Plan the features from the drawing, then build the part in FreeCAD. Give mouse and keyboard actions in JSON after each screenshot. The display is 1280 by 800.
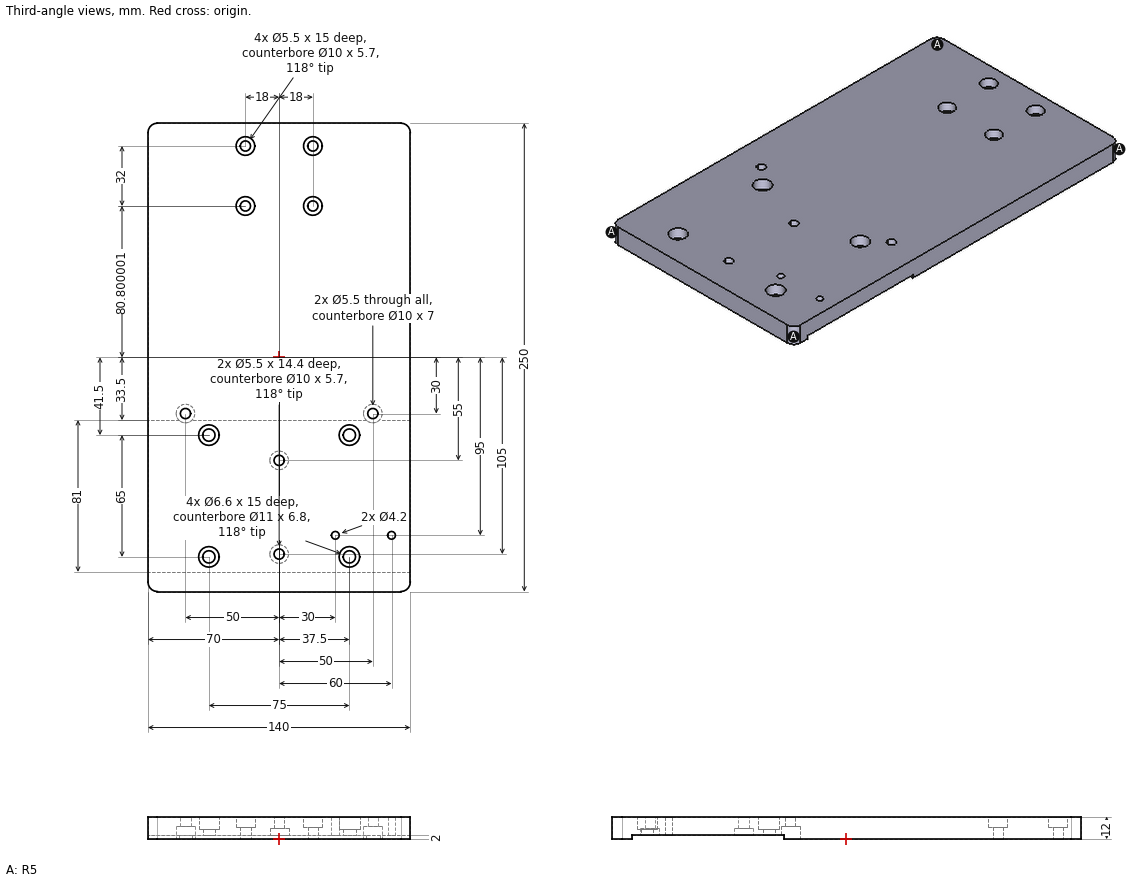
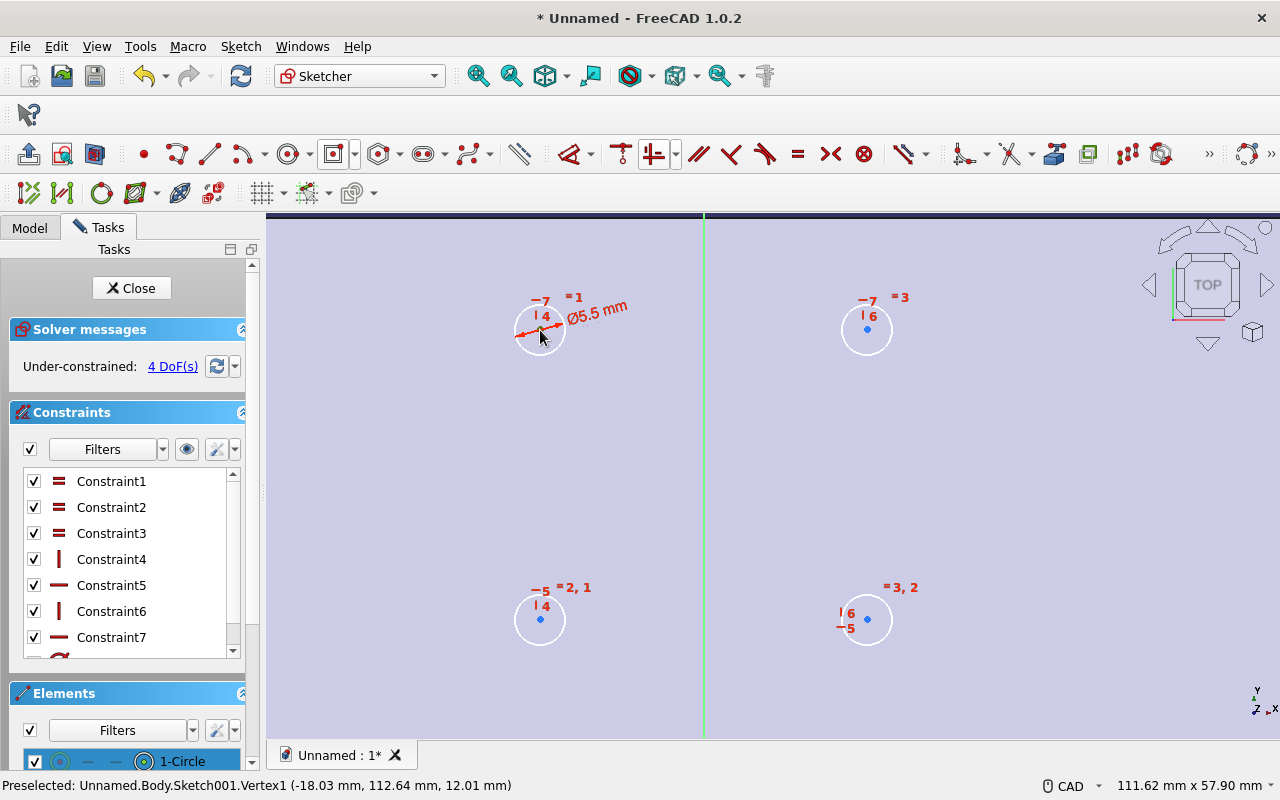
{"action": "key", "text": "l"}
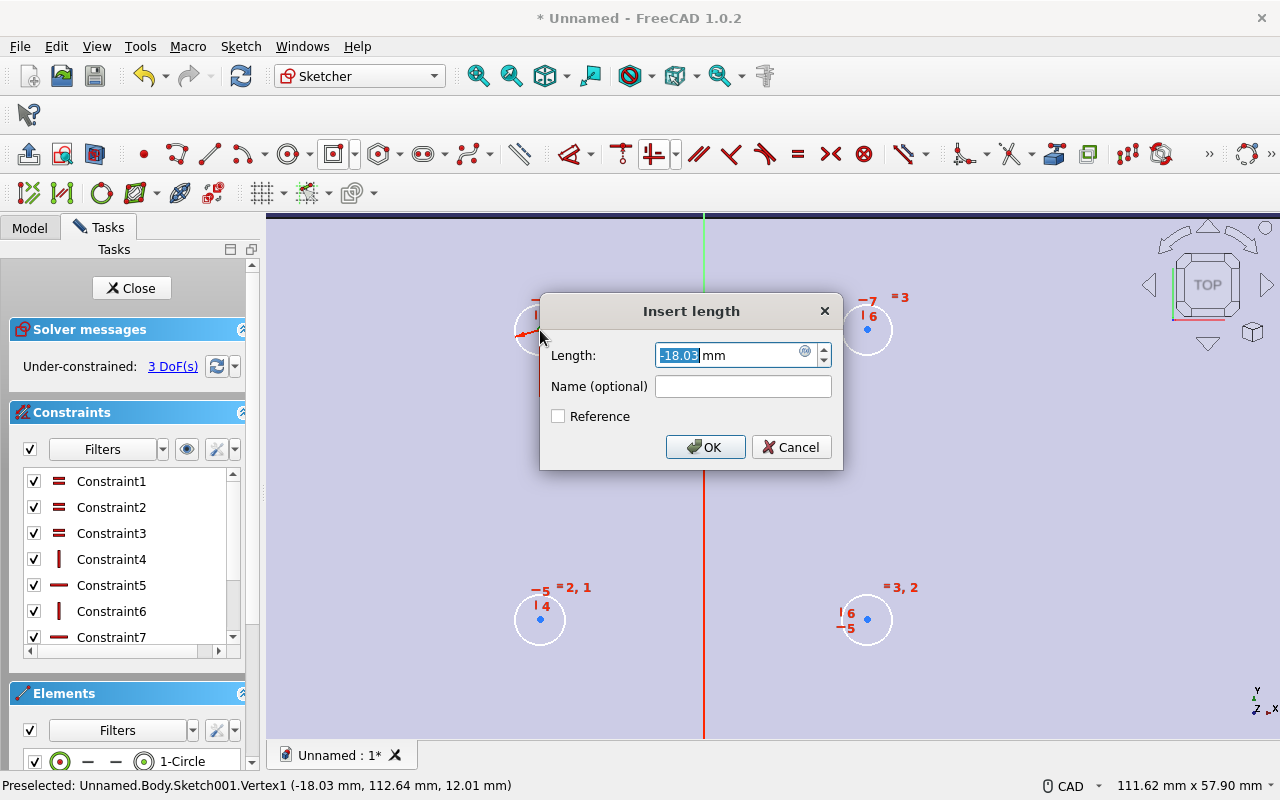
{"action": "type", "text": "-18"}
{"action": "key", "text": "Return"}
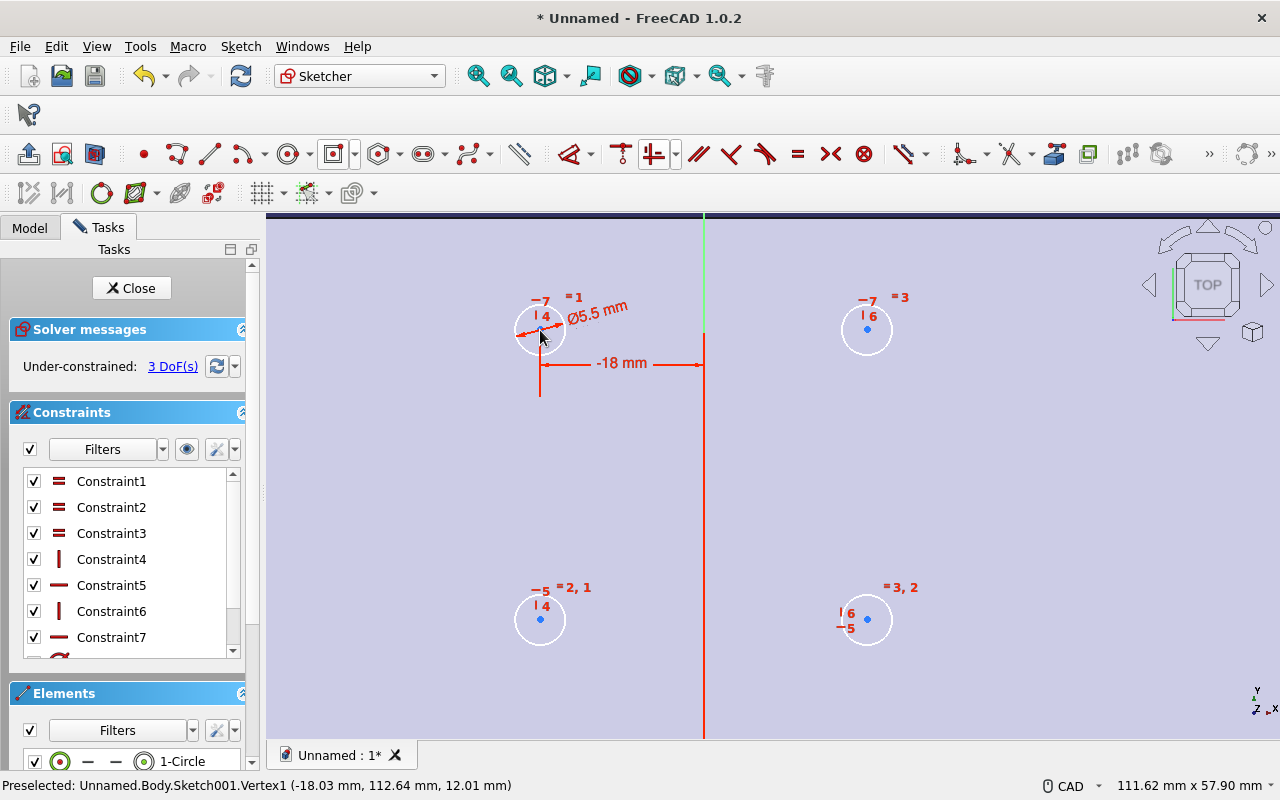
{"action": "left_click", "coordinate": [867, 620]}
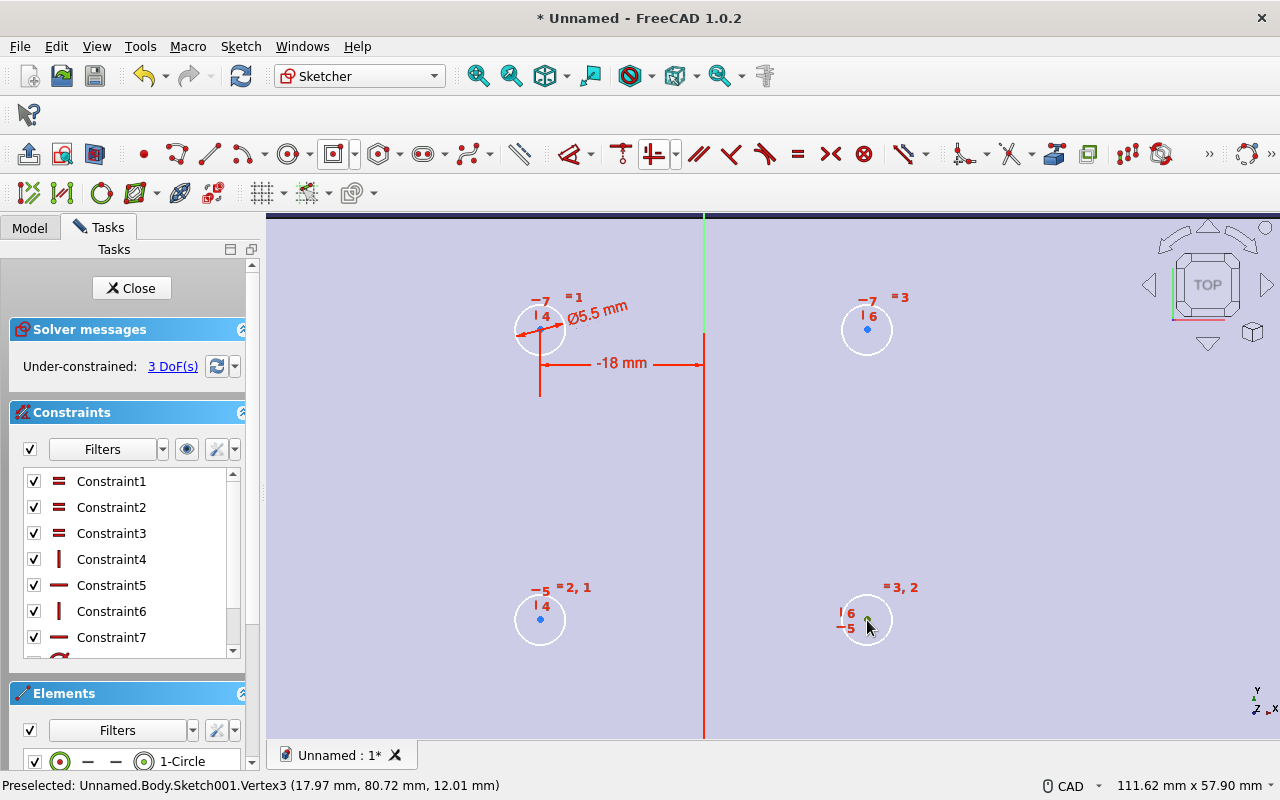
{"action": "key", "text": "l"}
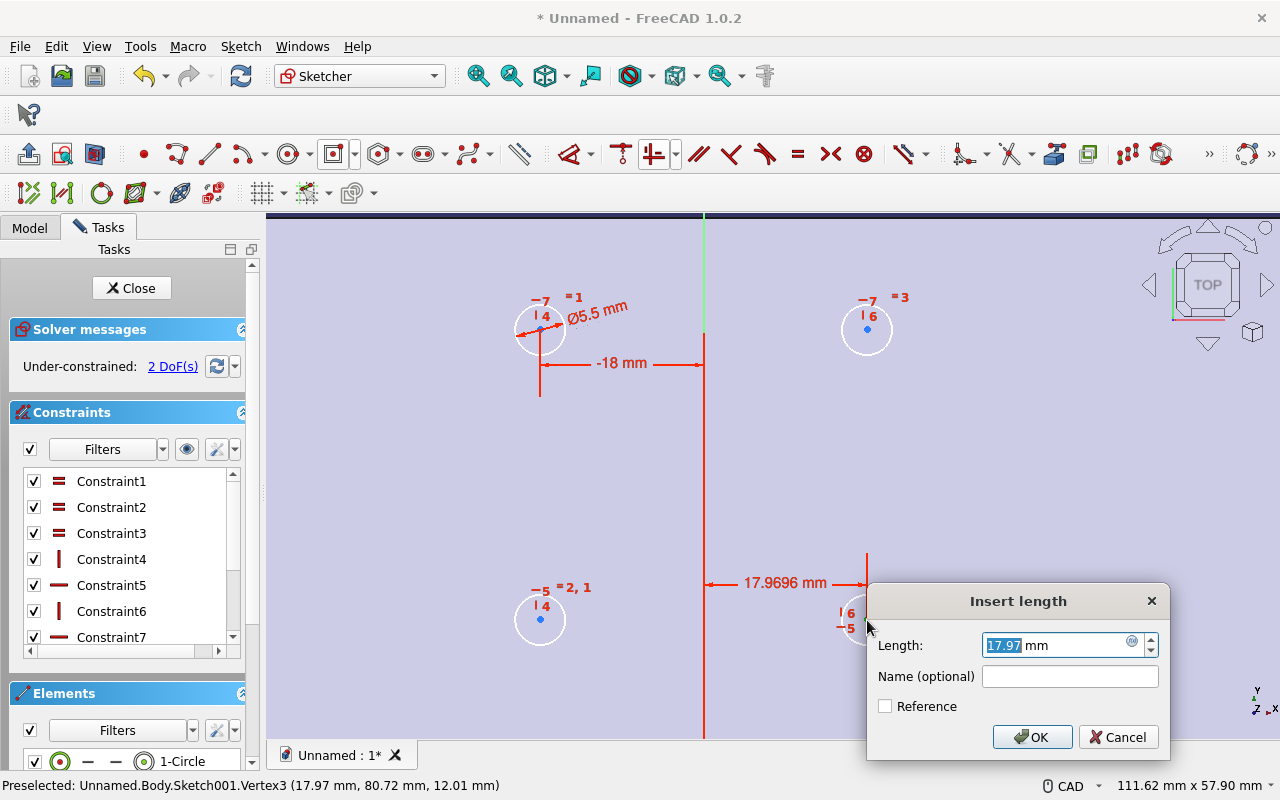
{"action": "type", "text": "18"}
{"action": "key", "text": "Return"}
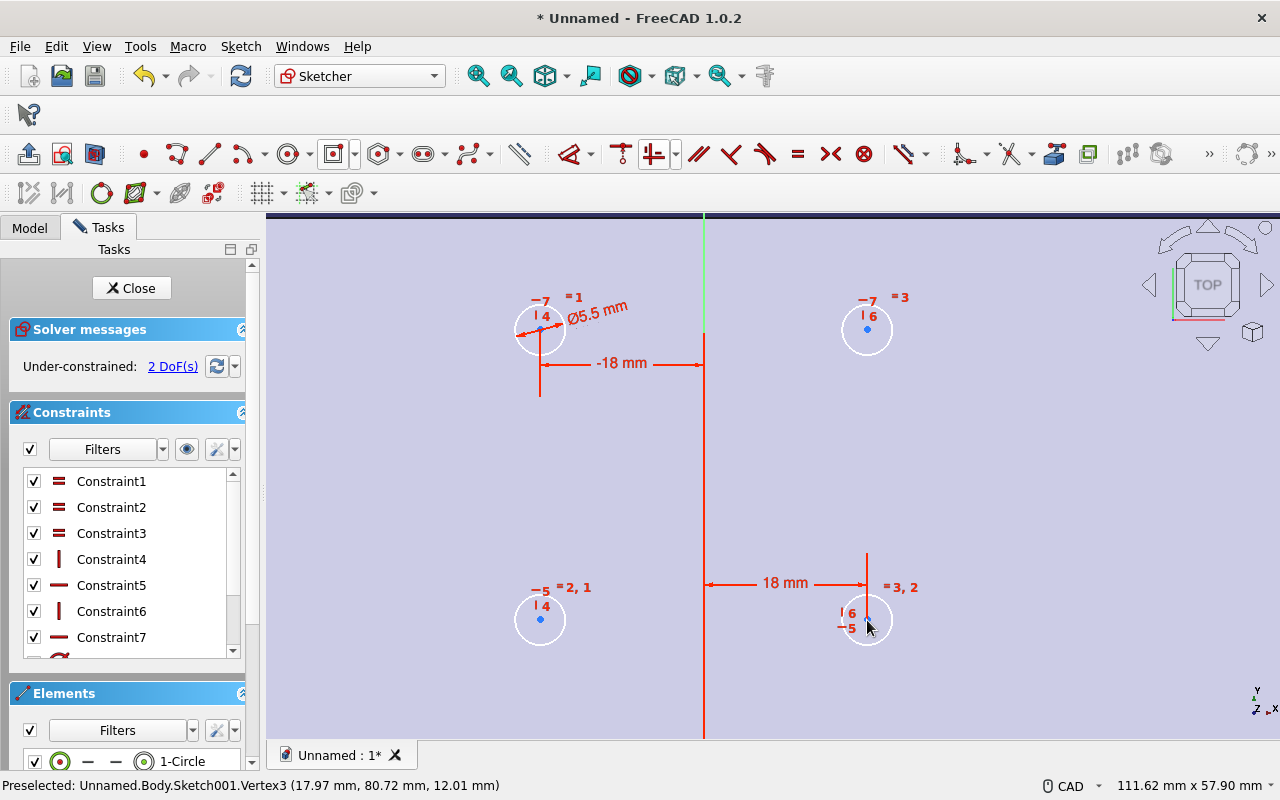
{"action": "left_click", "coordinate": [540, 330]}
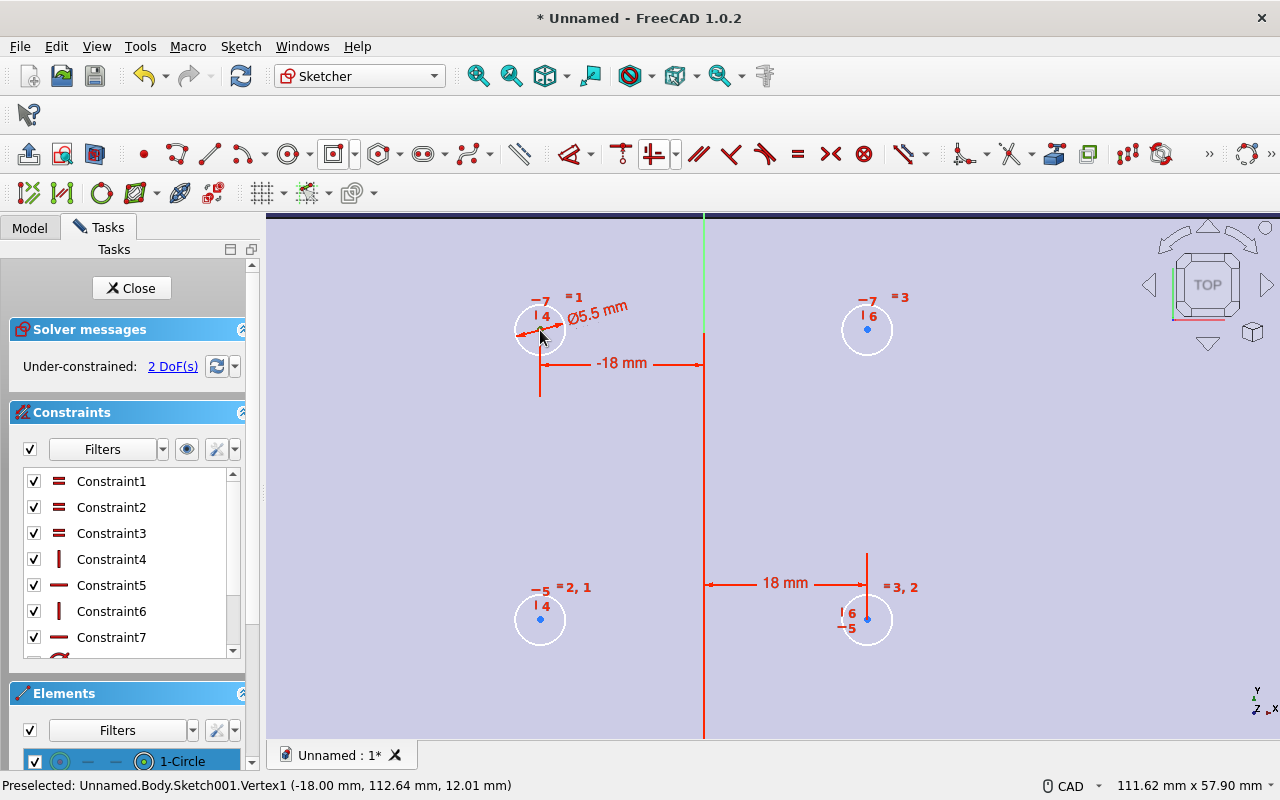
{"action": "left_click", "coordinate": [540, 620]}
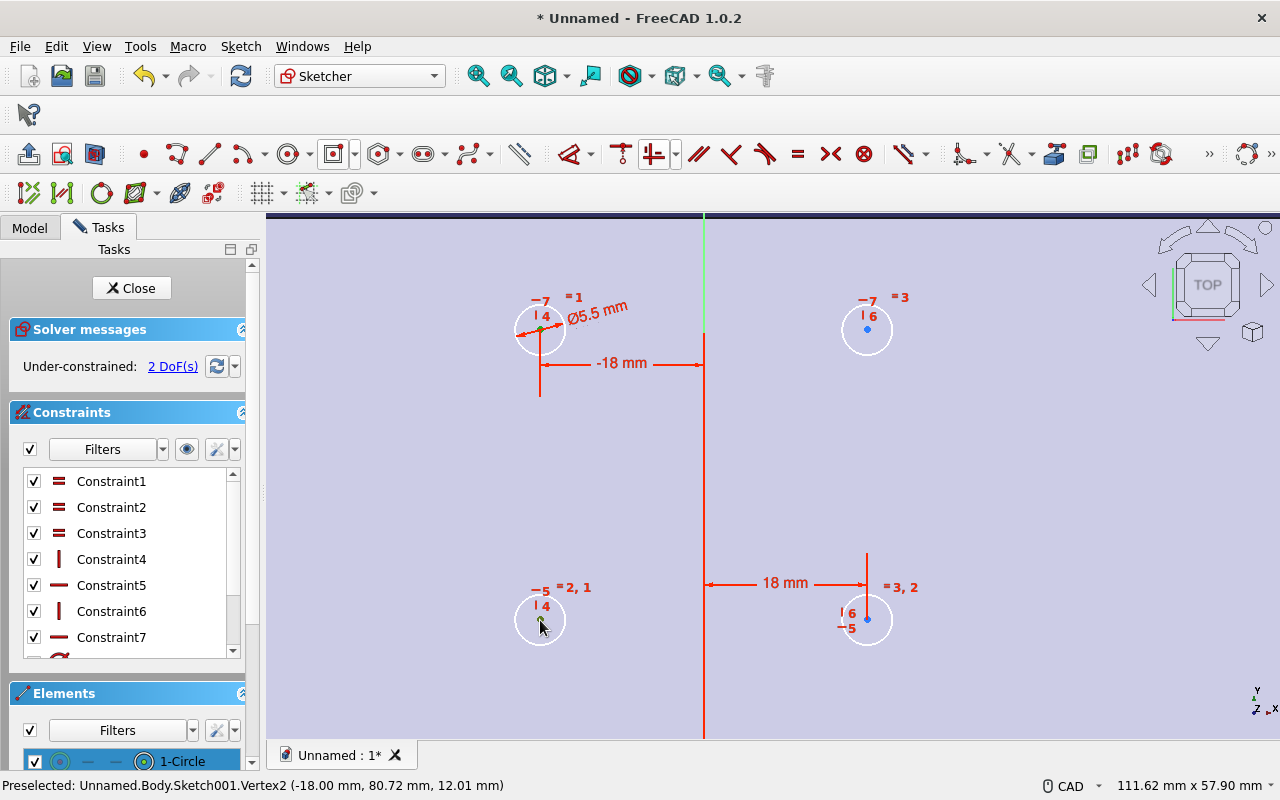
{"action": "key", "text": "i"}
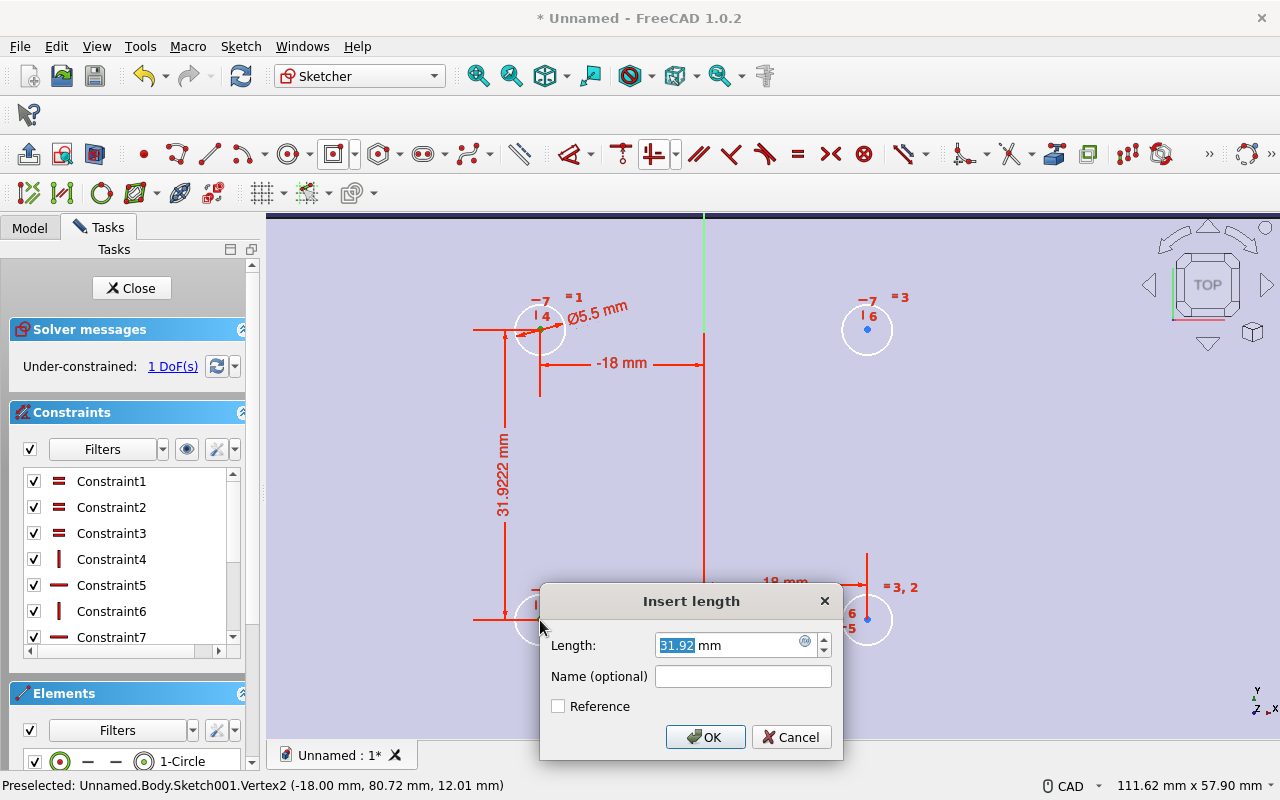
{"action": "type", "text": "32"}
{"action": "key", "text": "Return"}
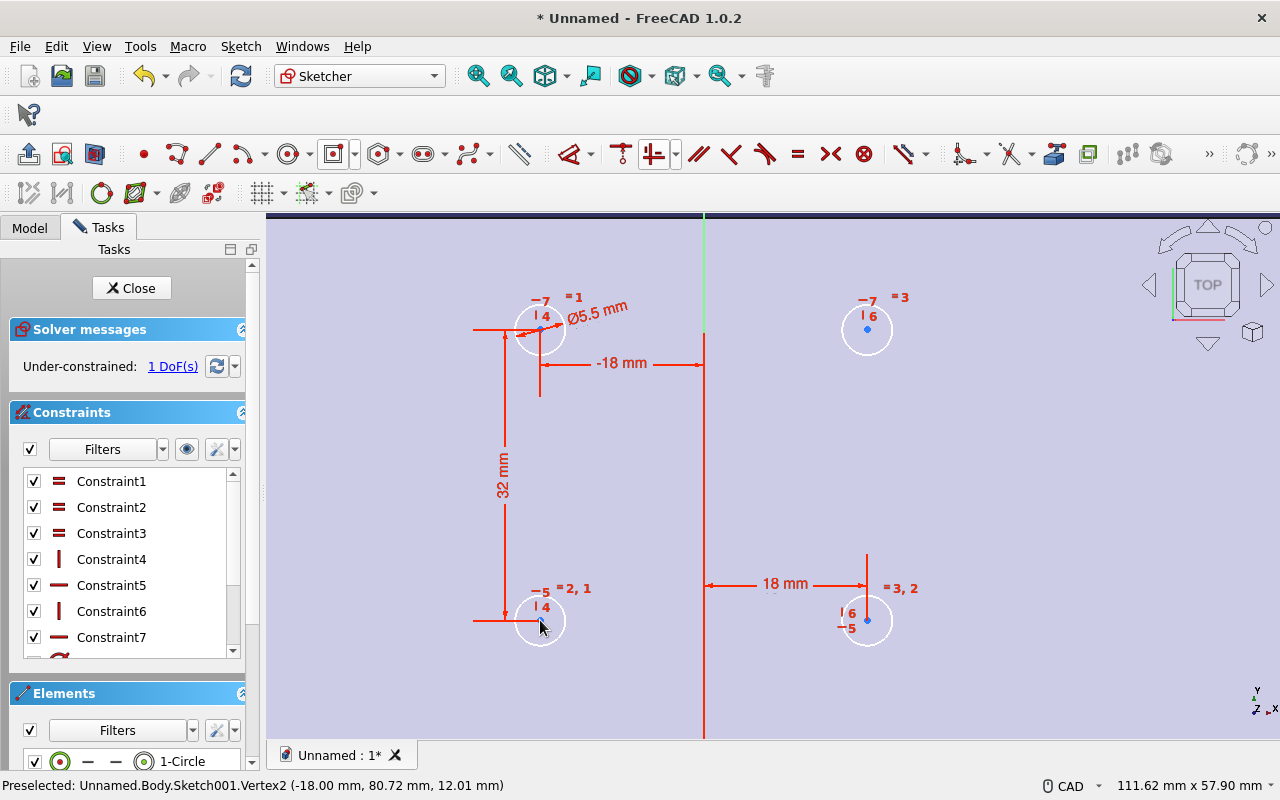
{"action": "left_click", "coordinate": [540, 621]}